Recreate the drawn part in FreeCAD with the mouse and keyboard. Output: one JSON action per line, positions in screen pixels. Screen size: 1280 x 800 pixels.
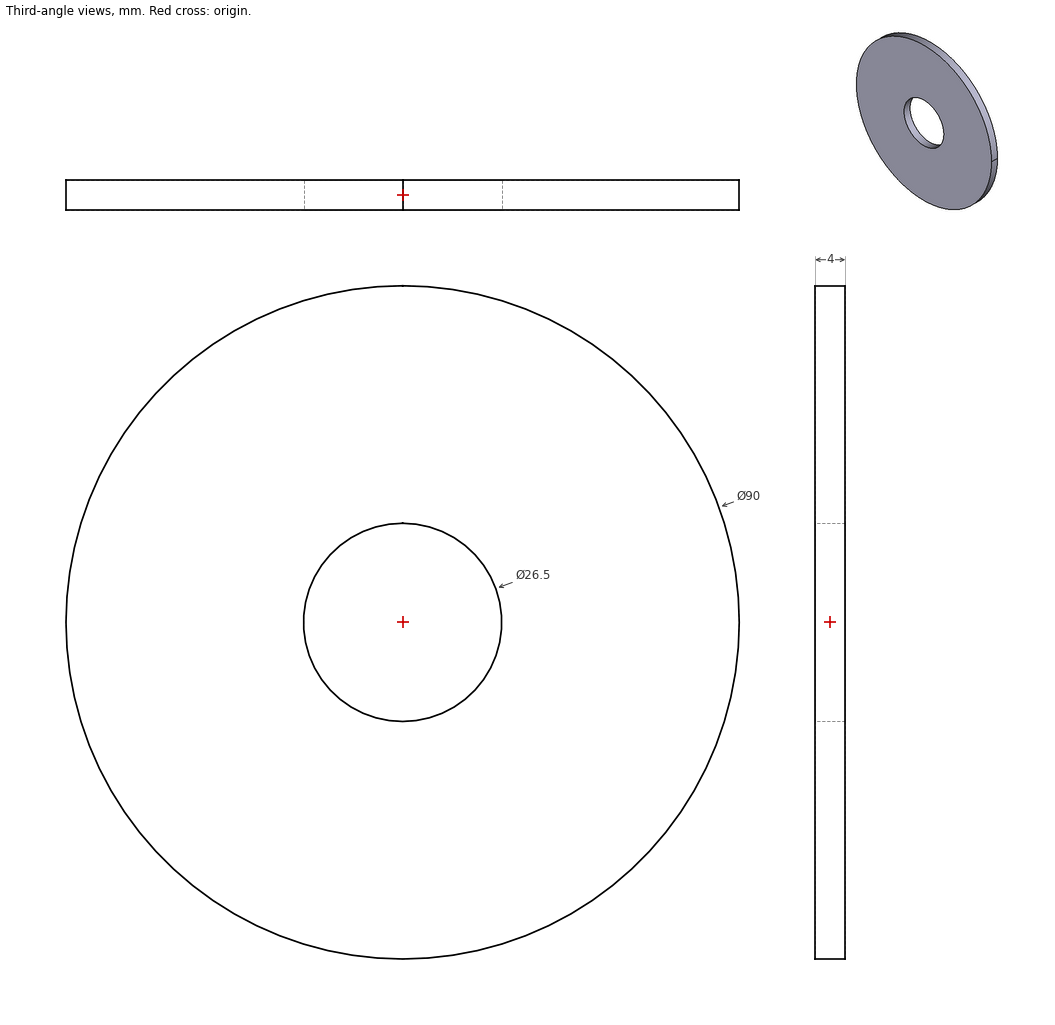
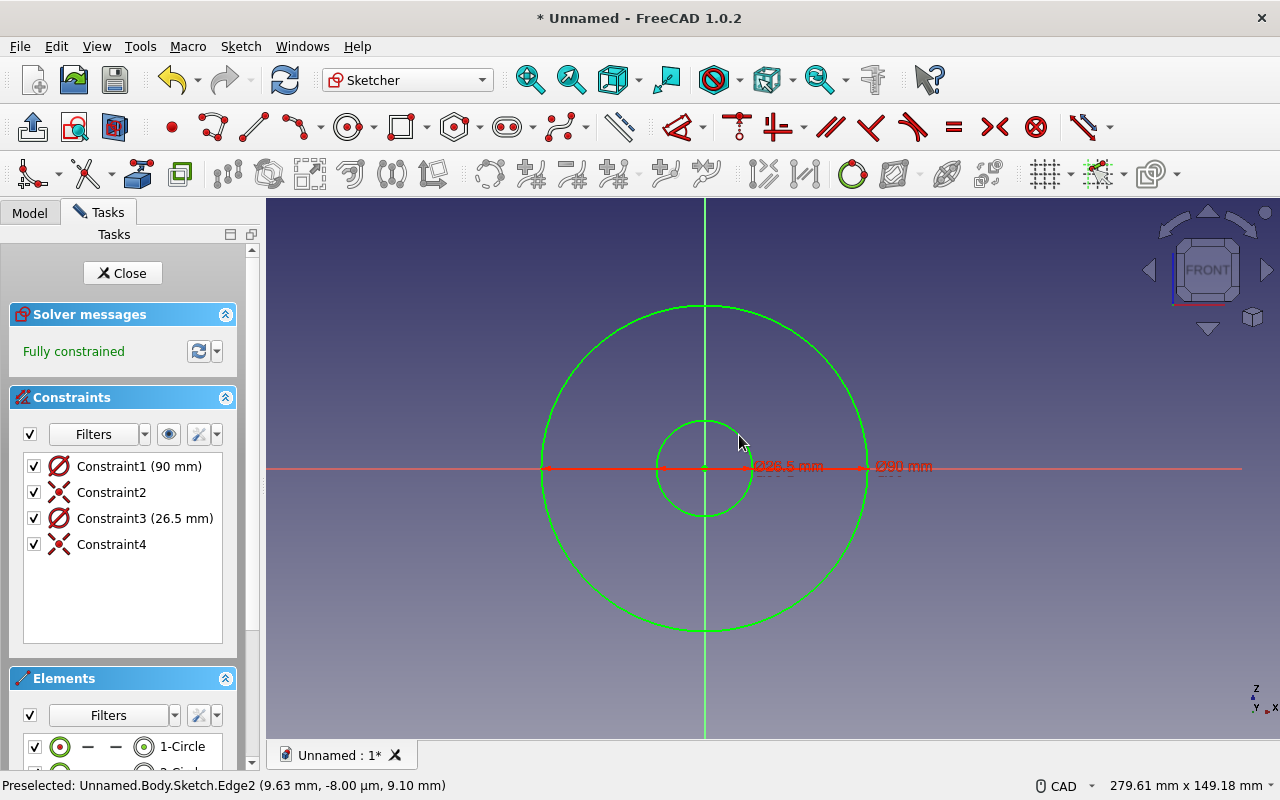
{"action": "left_click", "coordinate": [123, 273]}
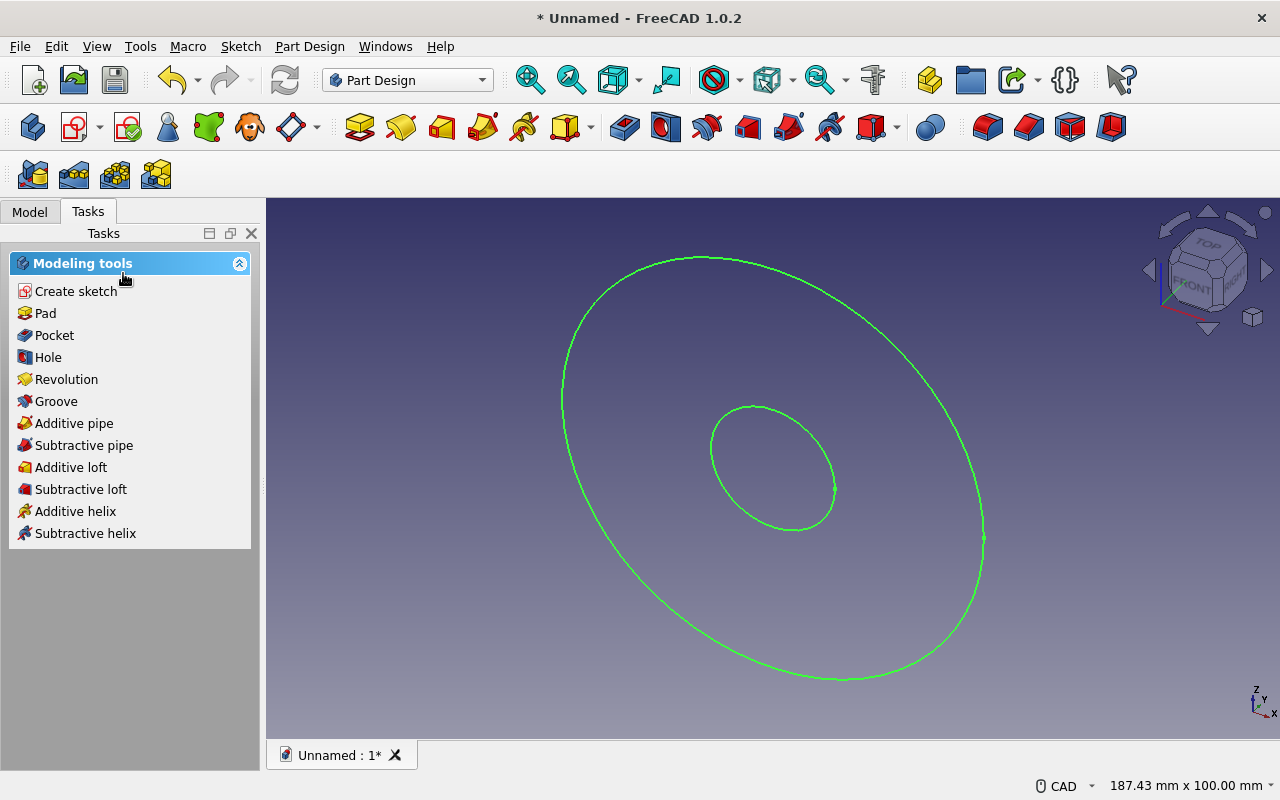
{"action": "left_click", "coordinate": [360, 128]}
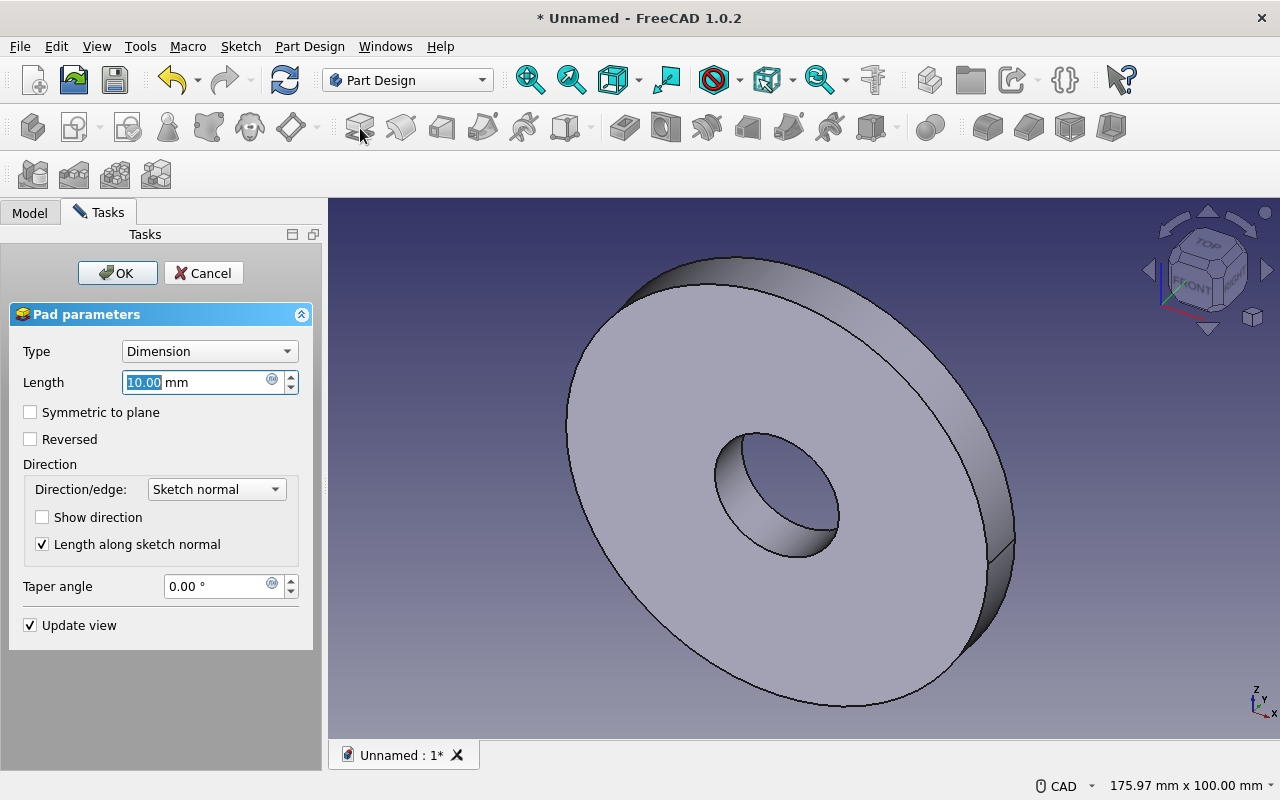
{"action": "type", "text": "4"}
{"action": "key", "text": "Tab"}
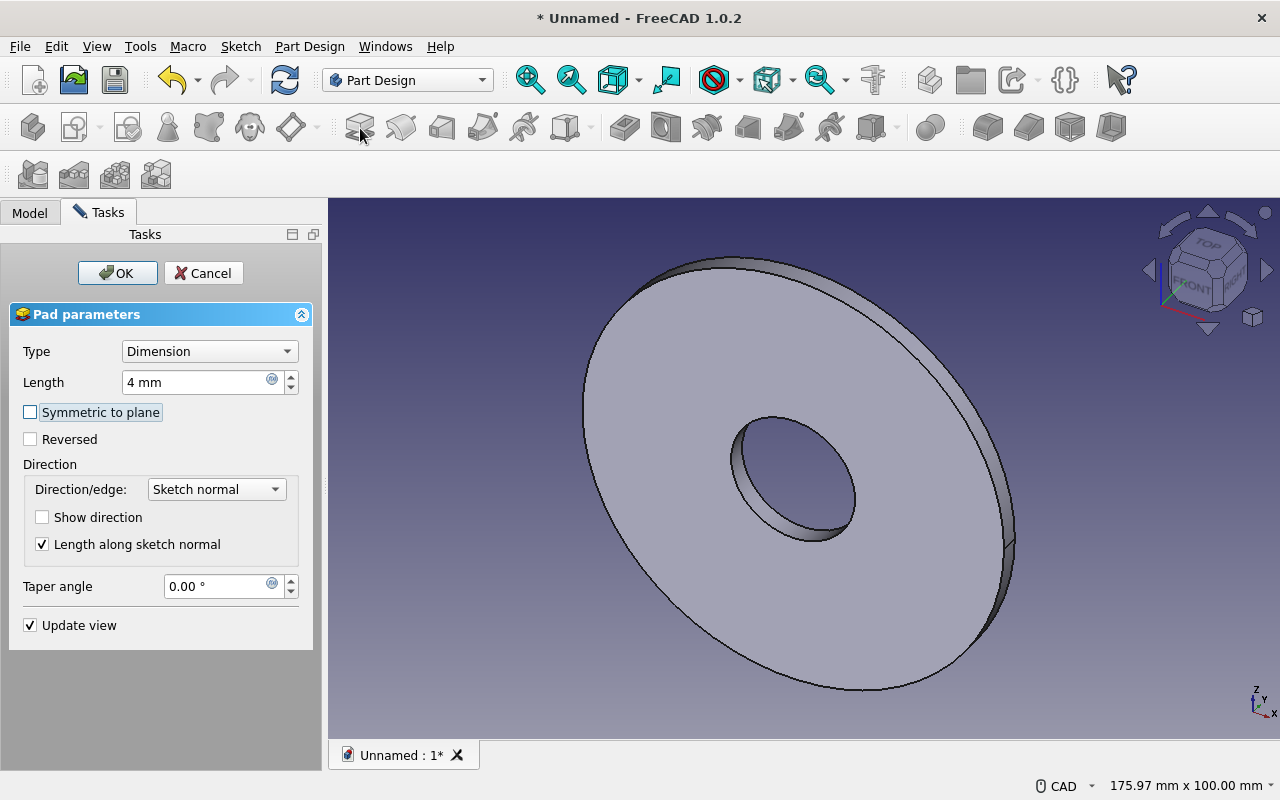
{"action": "left_click", "coordinate": [31, 412]}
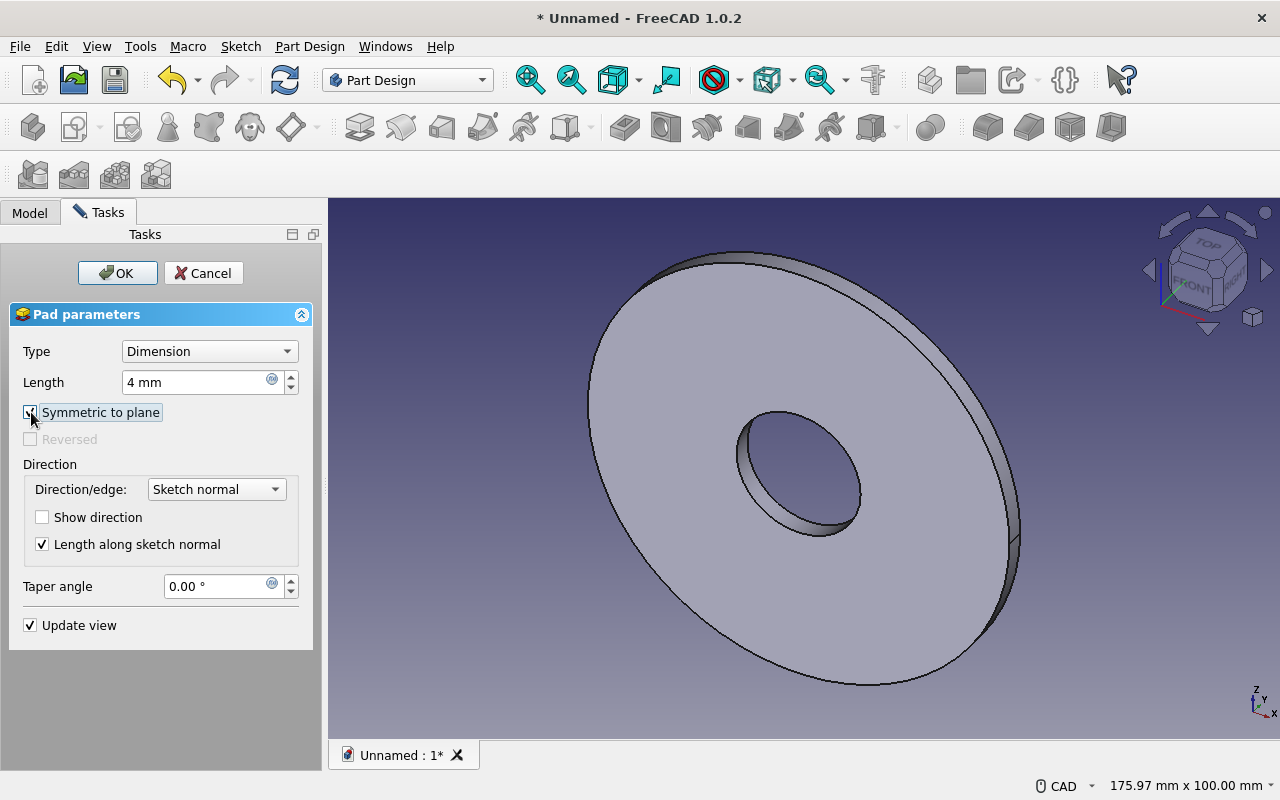
{"action": "left_click", "coordinate": [118, 273]}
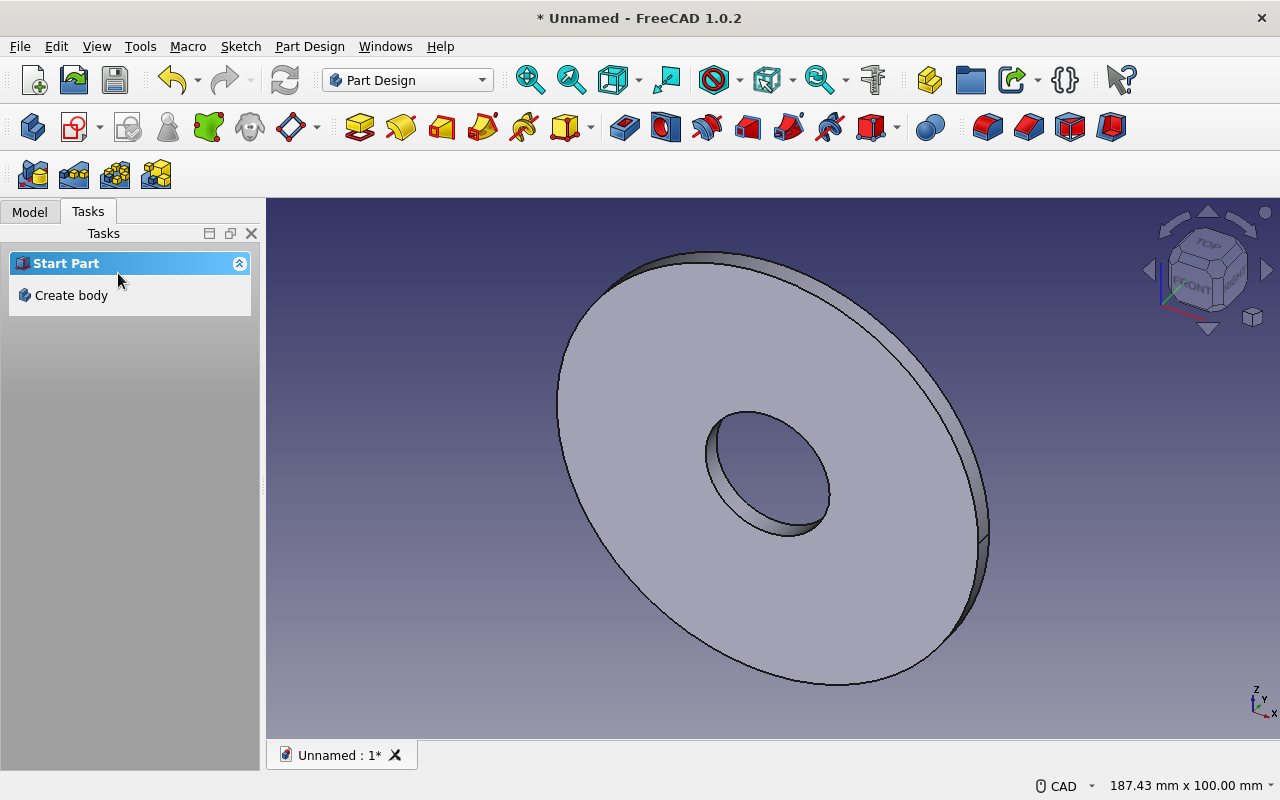
{"action": "key", "text": "0"}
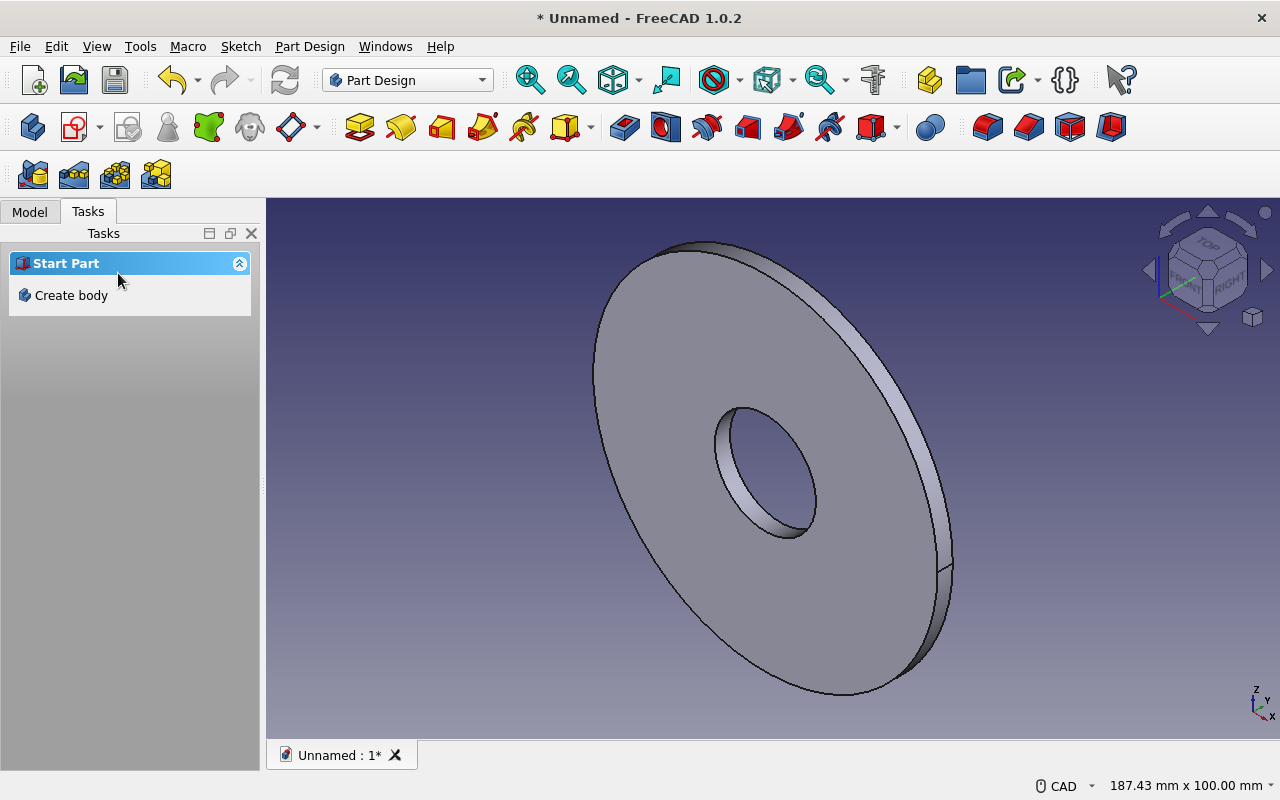
{"action": "key", "text": "v f"}